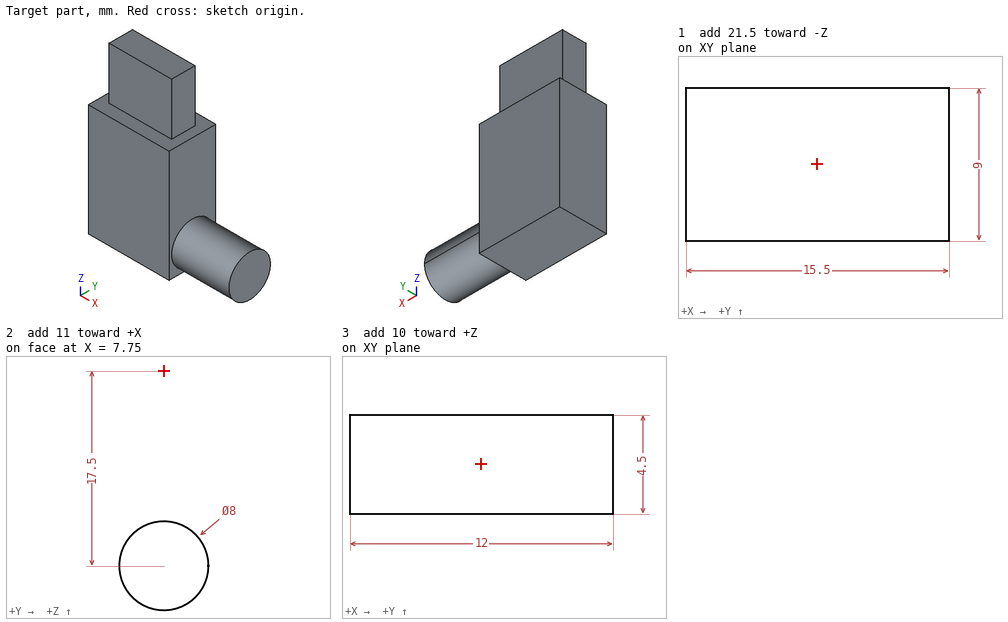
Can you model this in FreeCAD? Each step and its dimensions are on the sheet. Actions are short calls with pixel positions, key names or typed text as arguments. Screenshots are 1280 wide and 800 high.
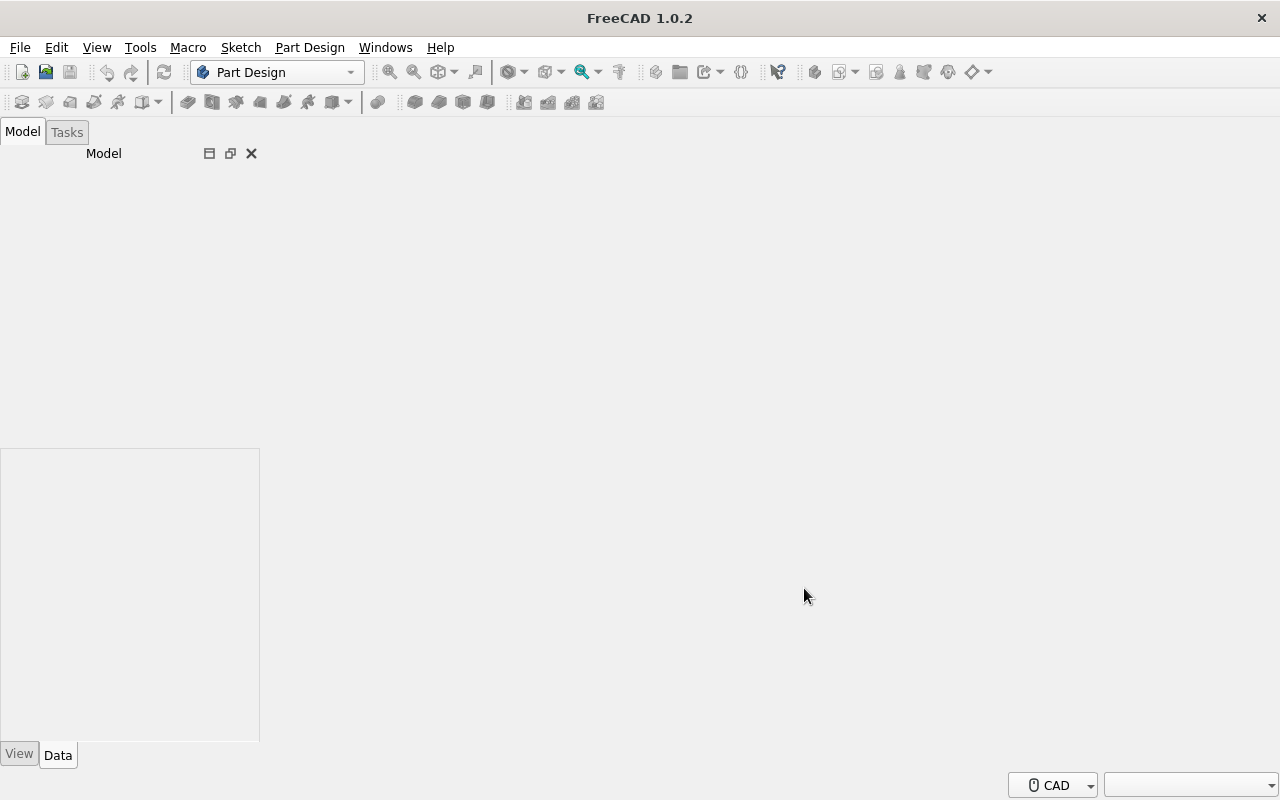
click(22, 72)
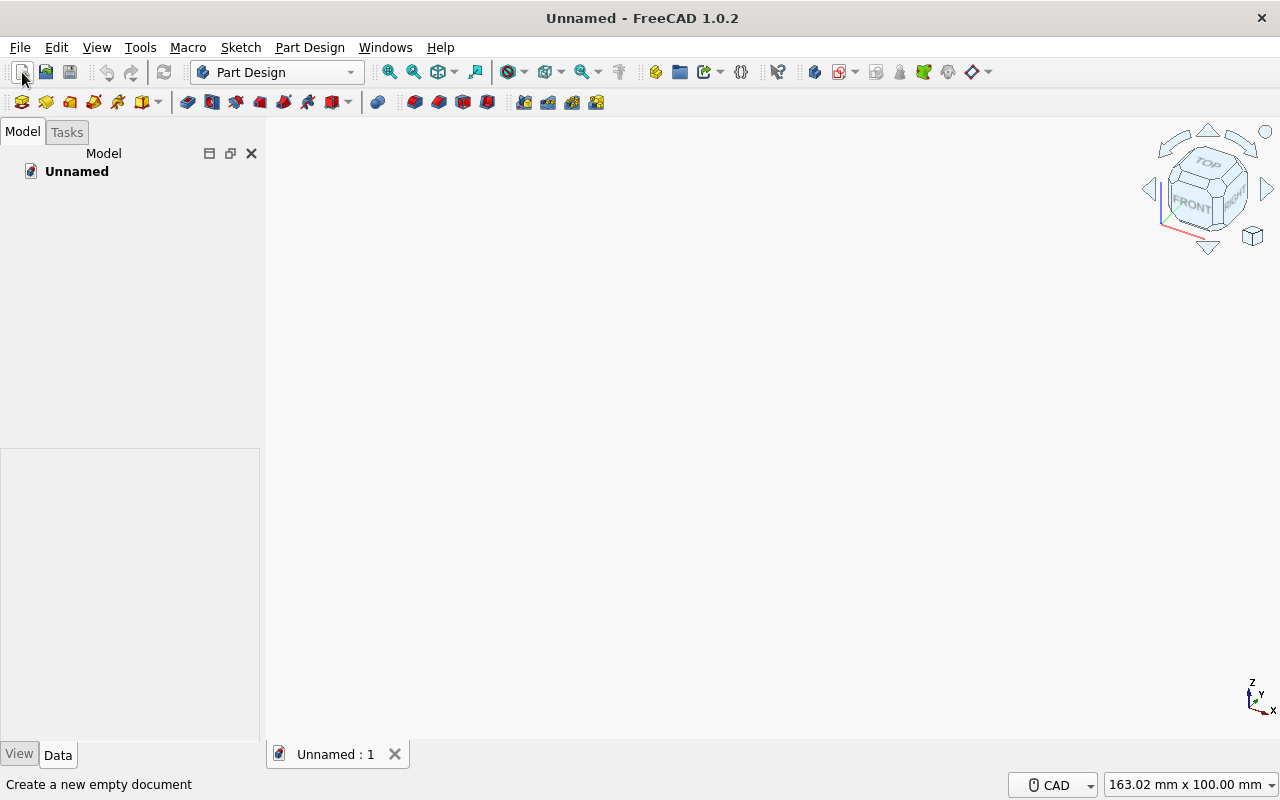
click(840, 72)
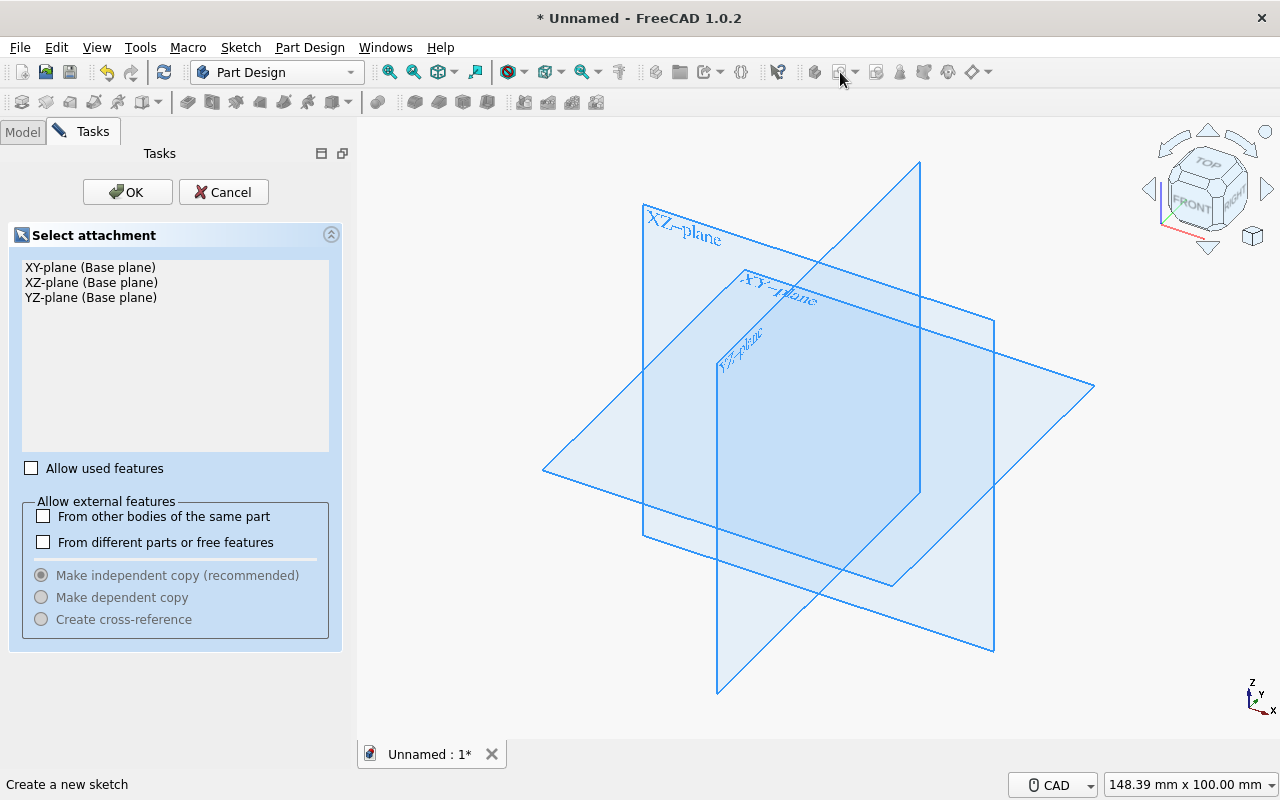
click(82, 268)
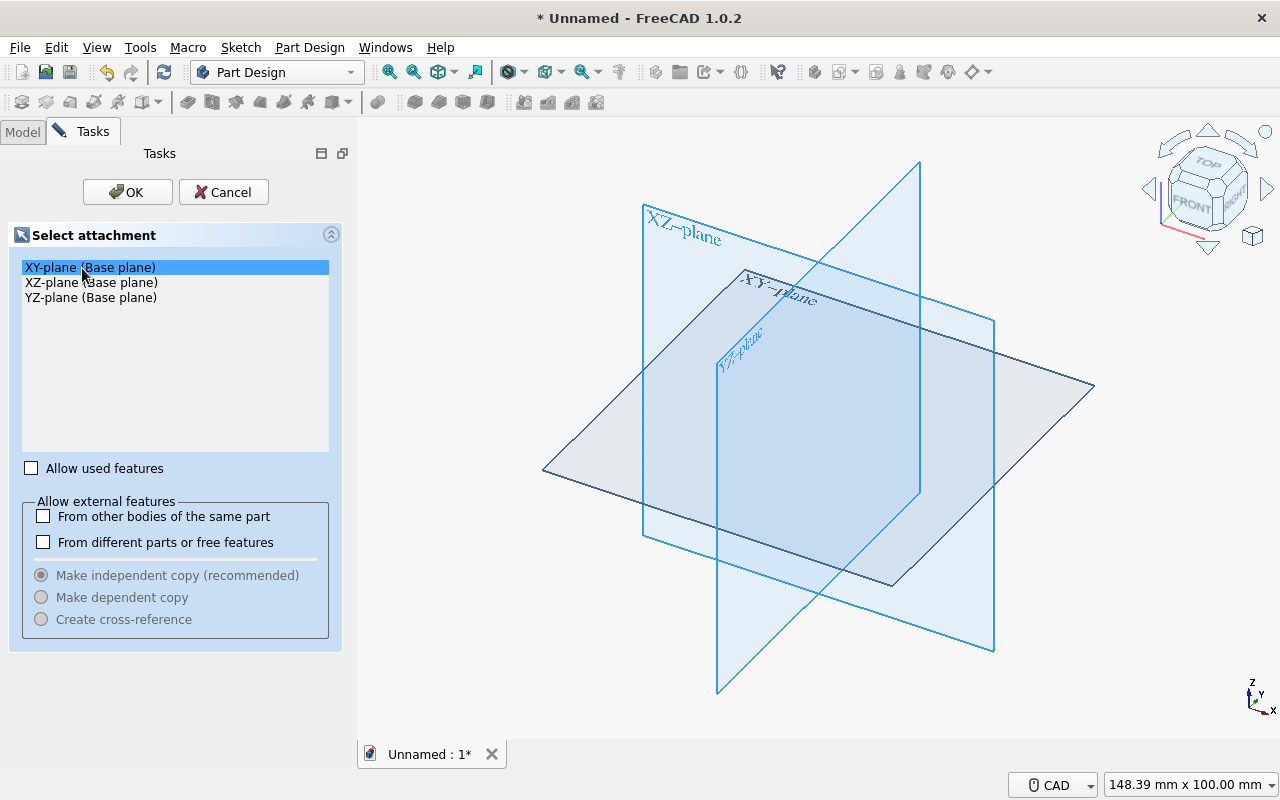
click(128, 192)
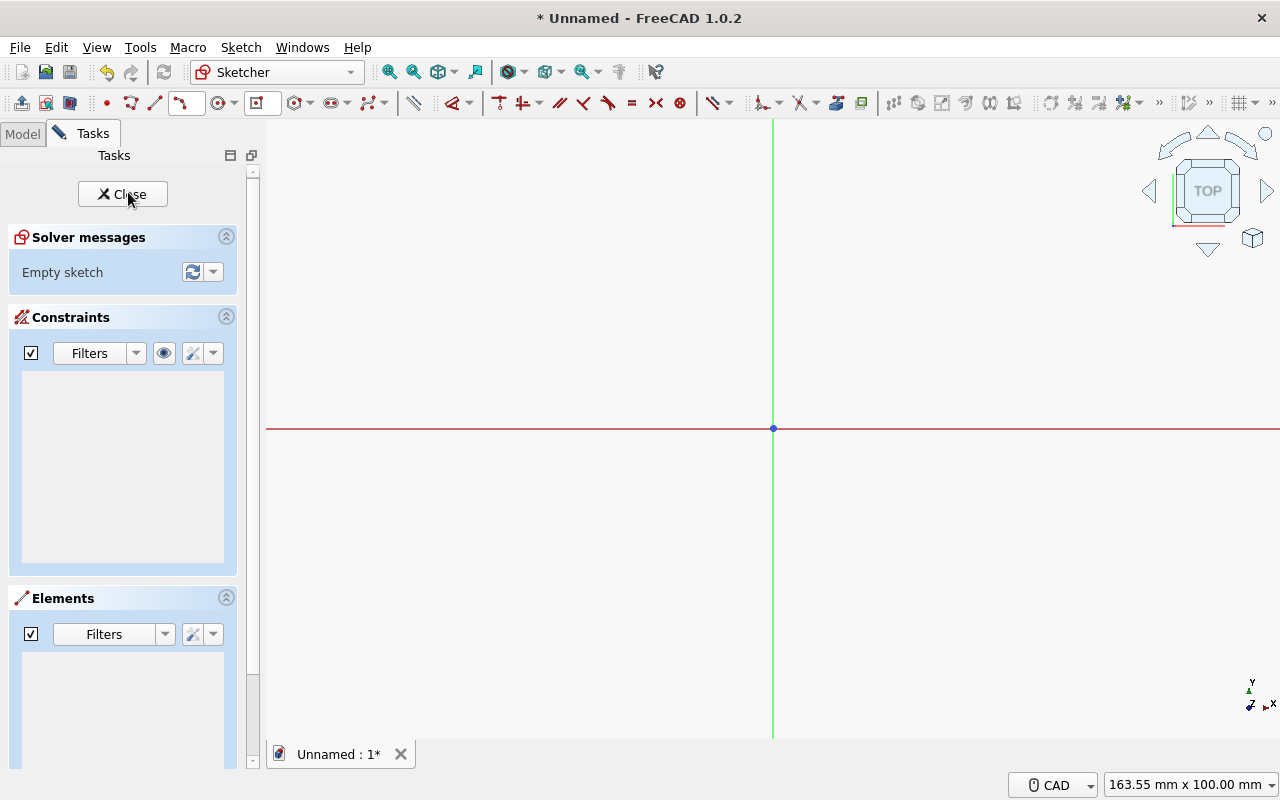
scroll(787, 429, up, 9)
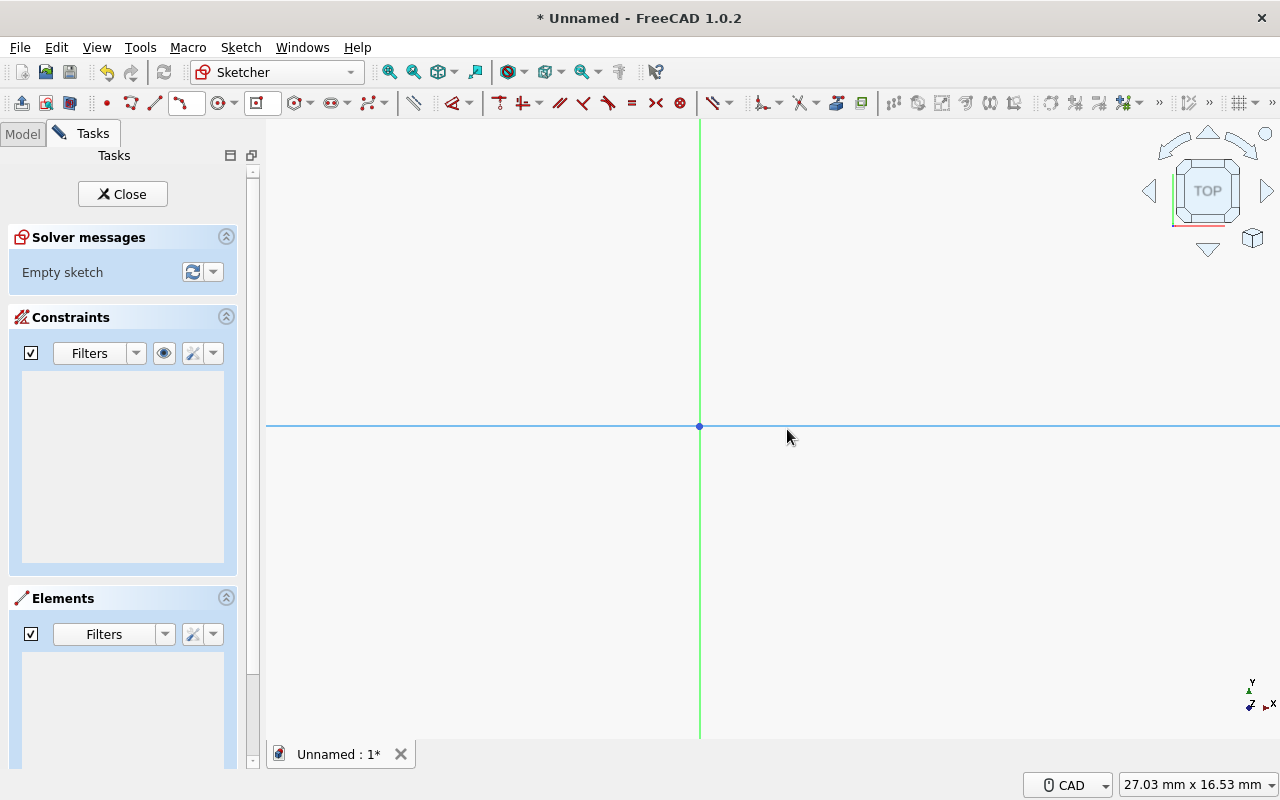
click(256, 104)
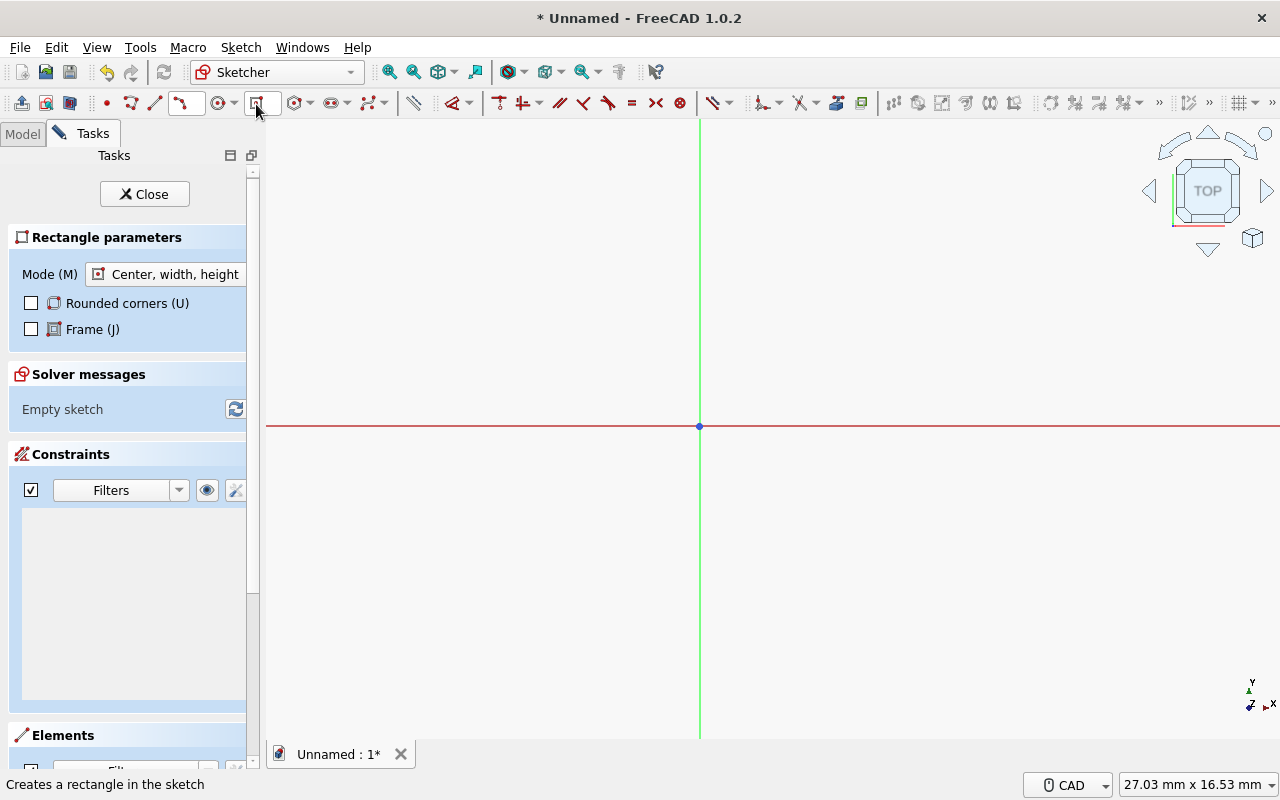
click(700, 426)
move(990, 258)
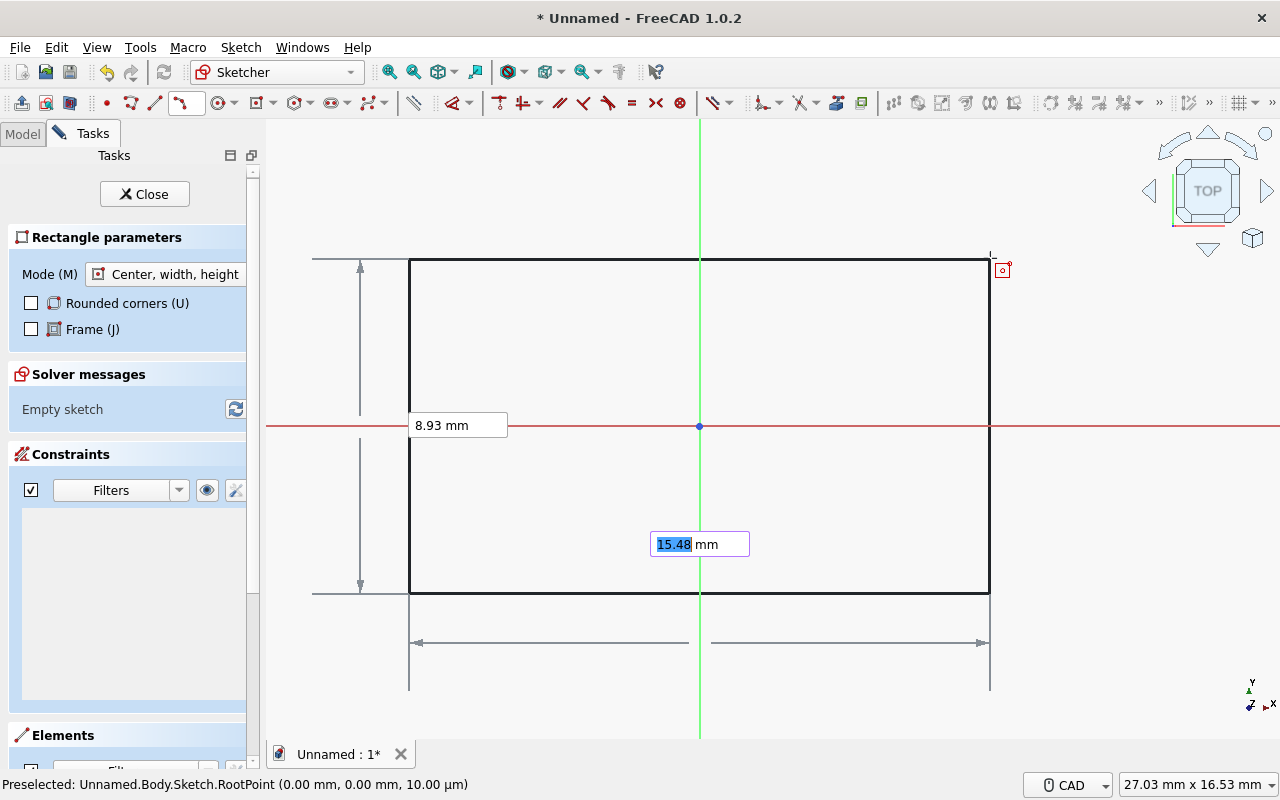
text(15.5)
key(Tab)
text(9)
key(Return)
key(Escape)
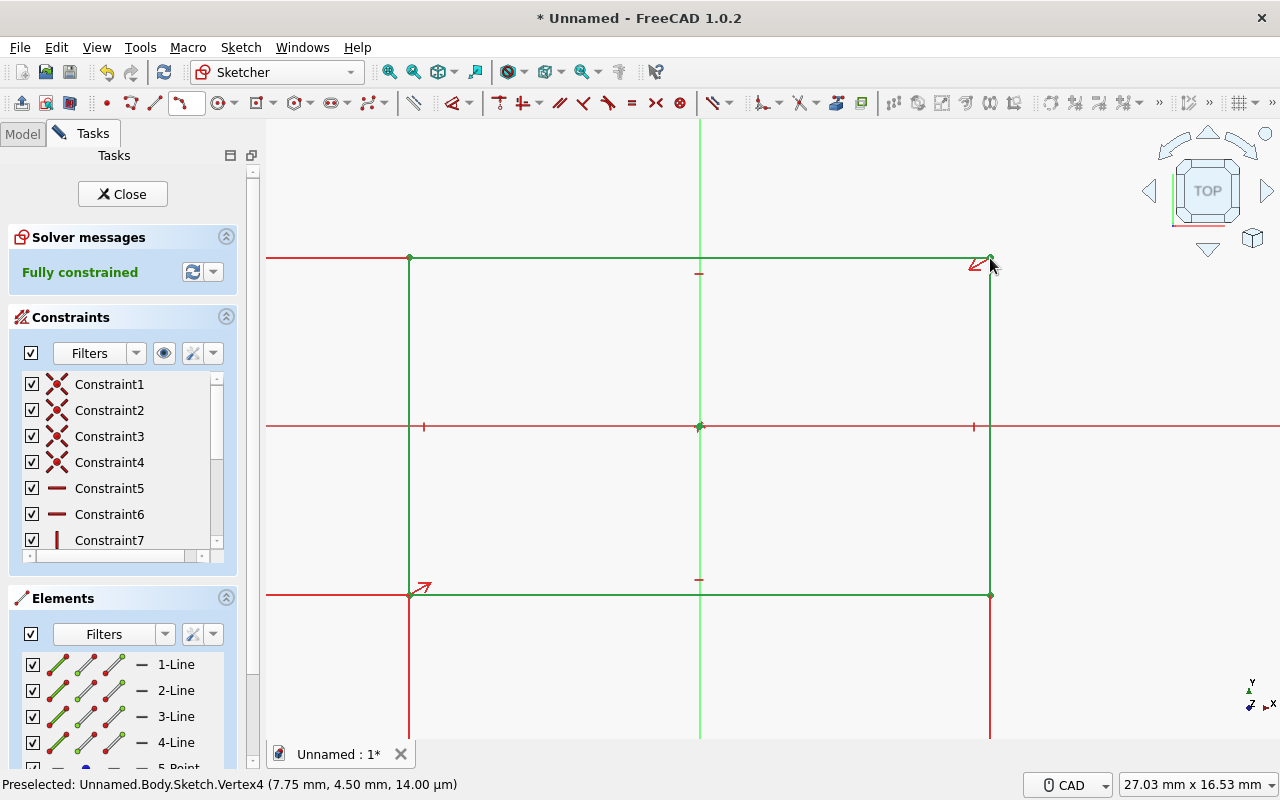
click(123, 194)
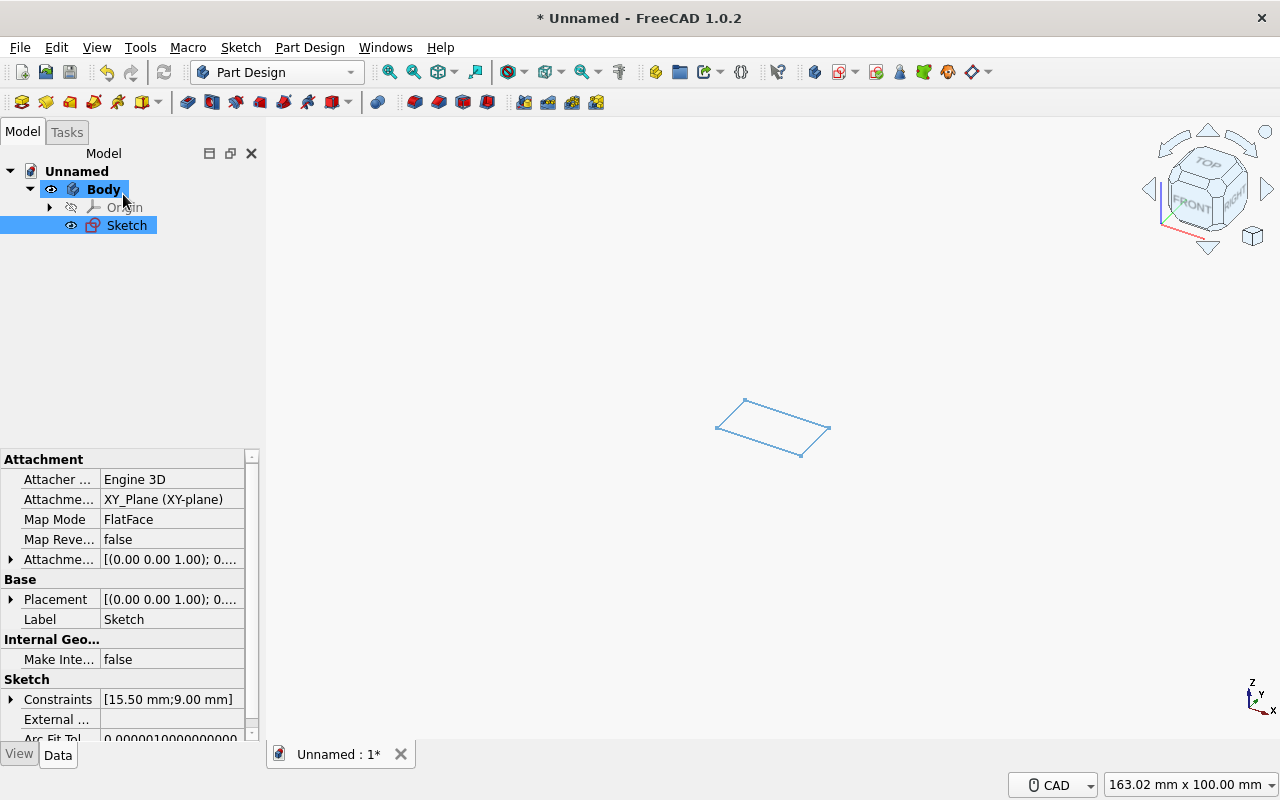
click(22, 102)